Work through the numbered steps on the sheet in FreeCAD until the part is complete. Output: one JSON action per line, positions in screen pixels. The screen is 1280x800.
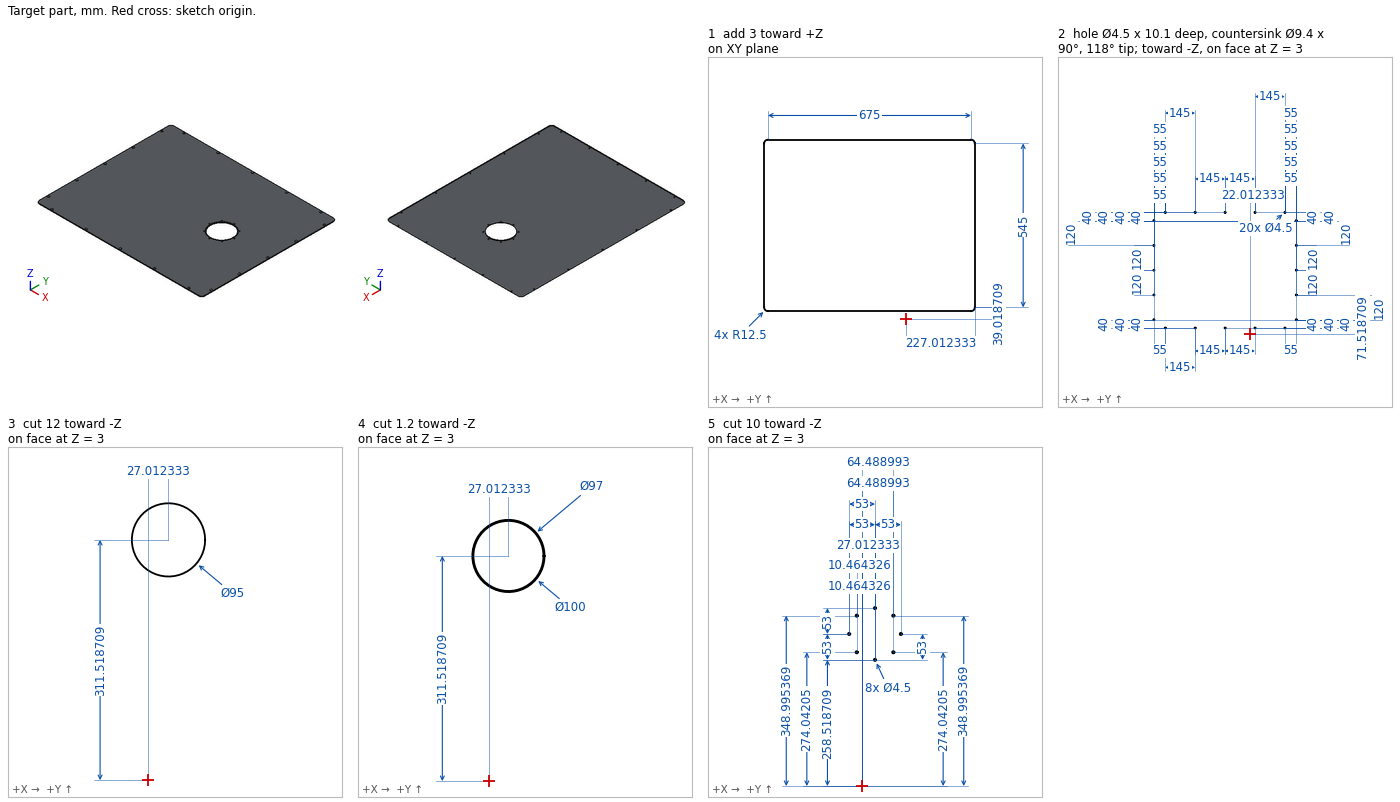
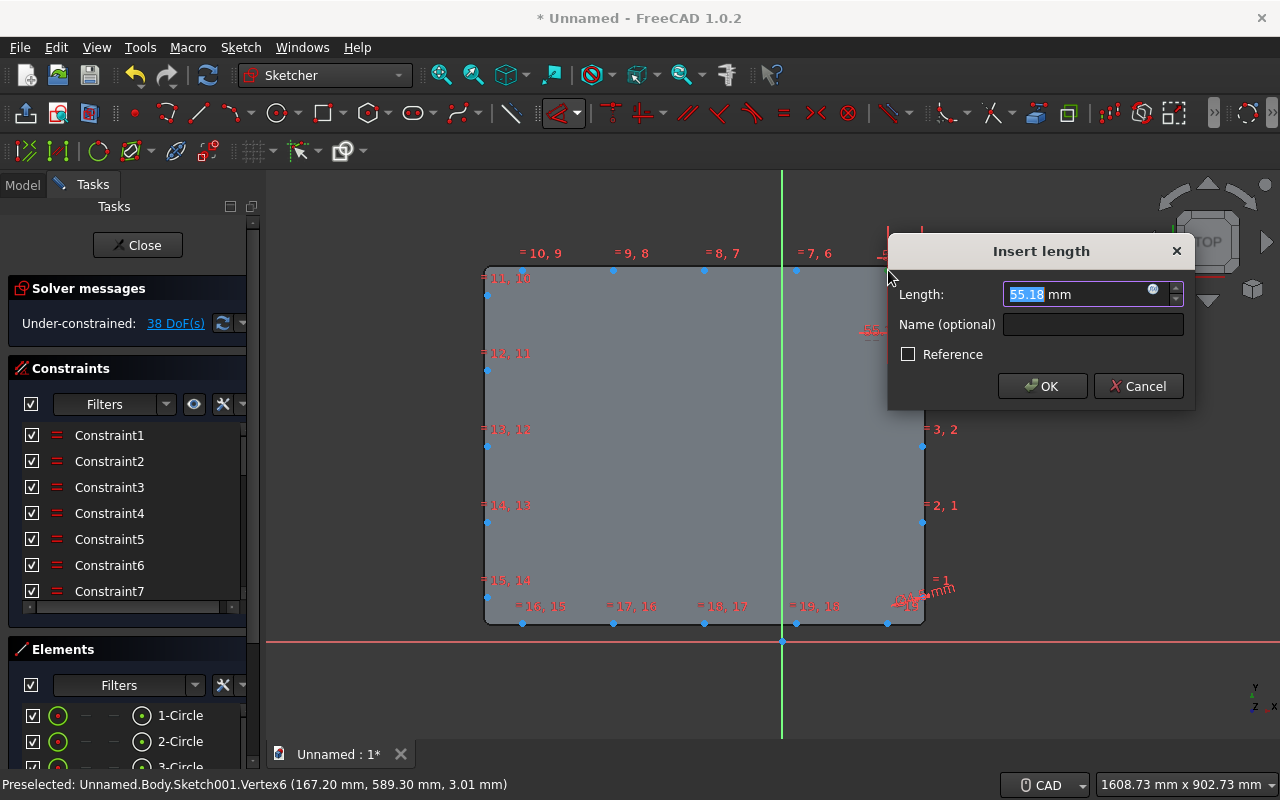
{"action": "type", "text": "55"}
{"action": "key", "text": "Return"}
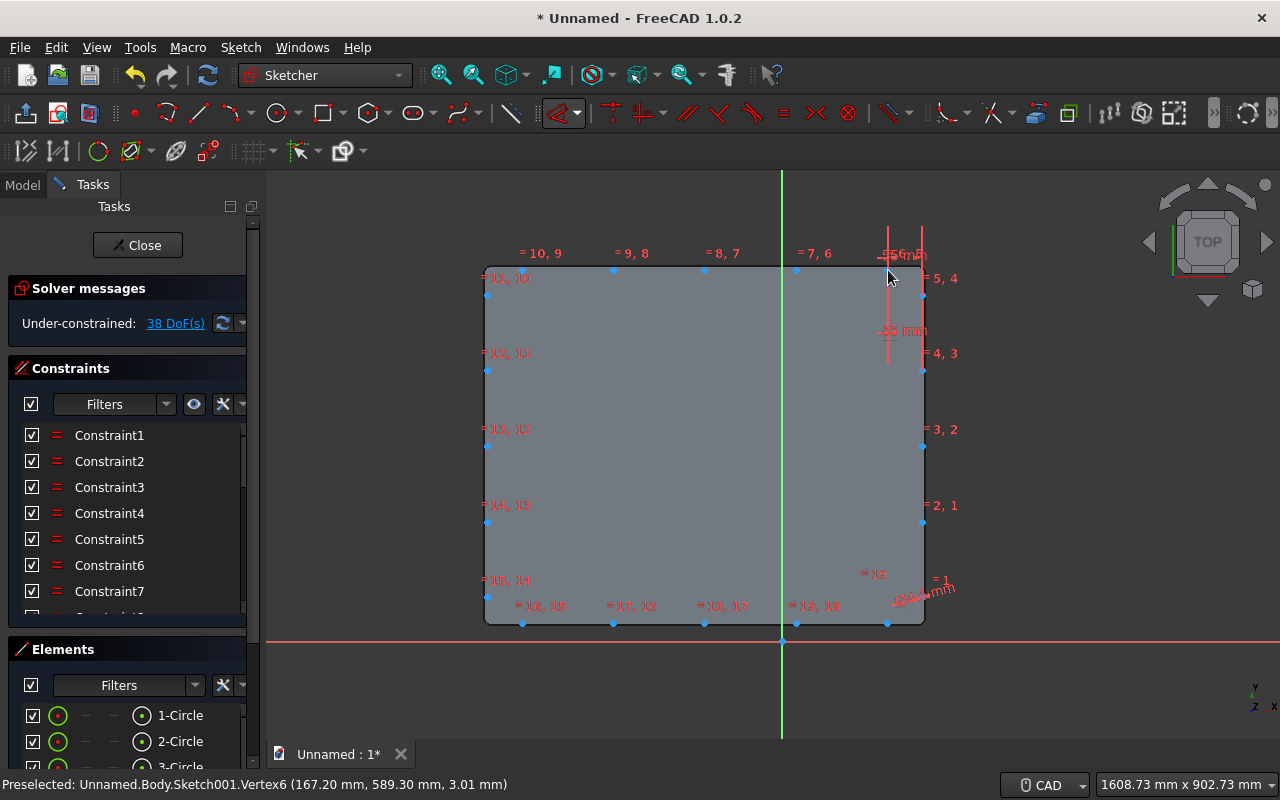
{"action": "left_click", "coordinate": [922, 446]}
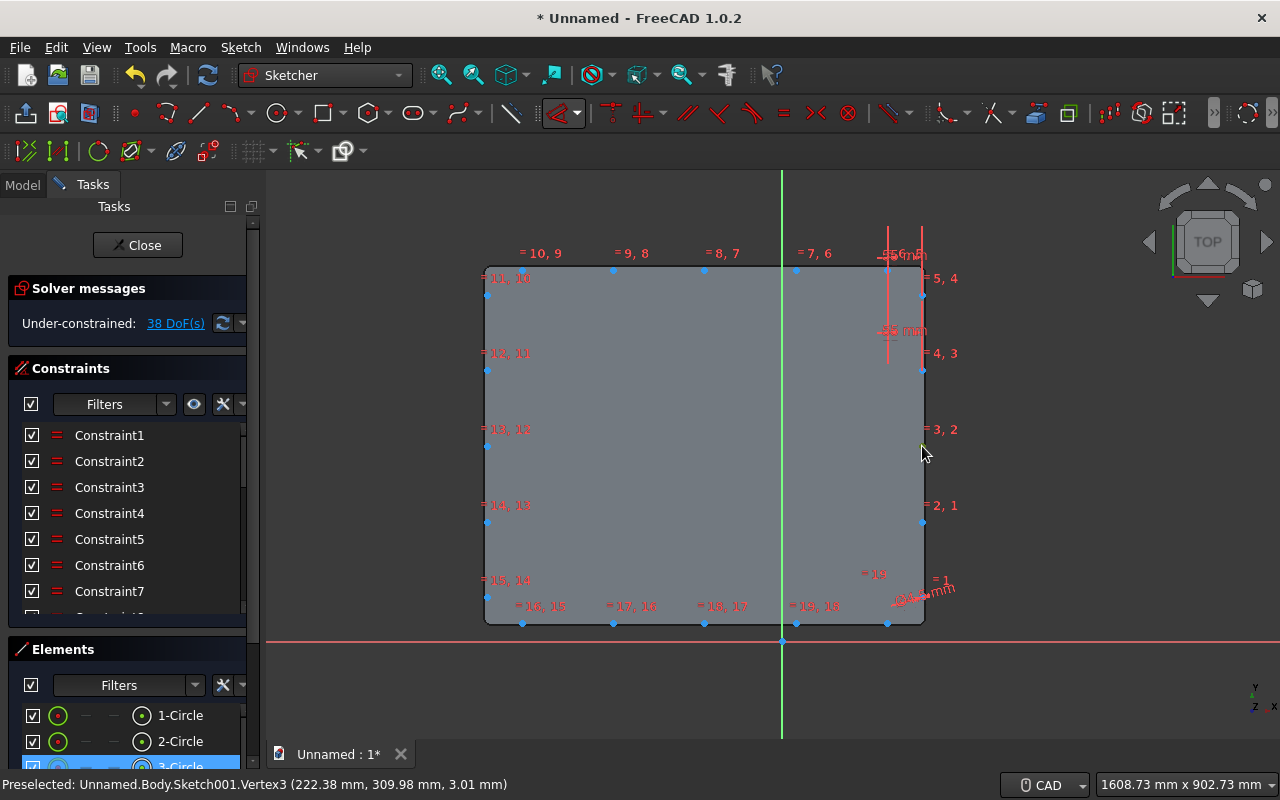
{"action": "left_click", "coordinate": [888, 270]}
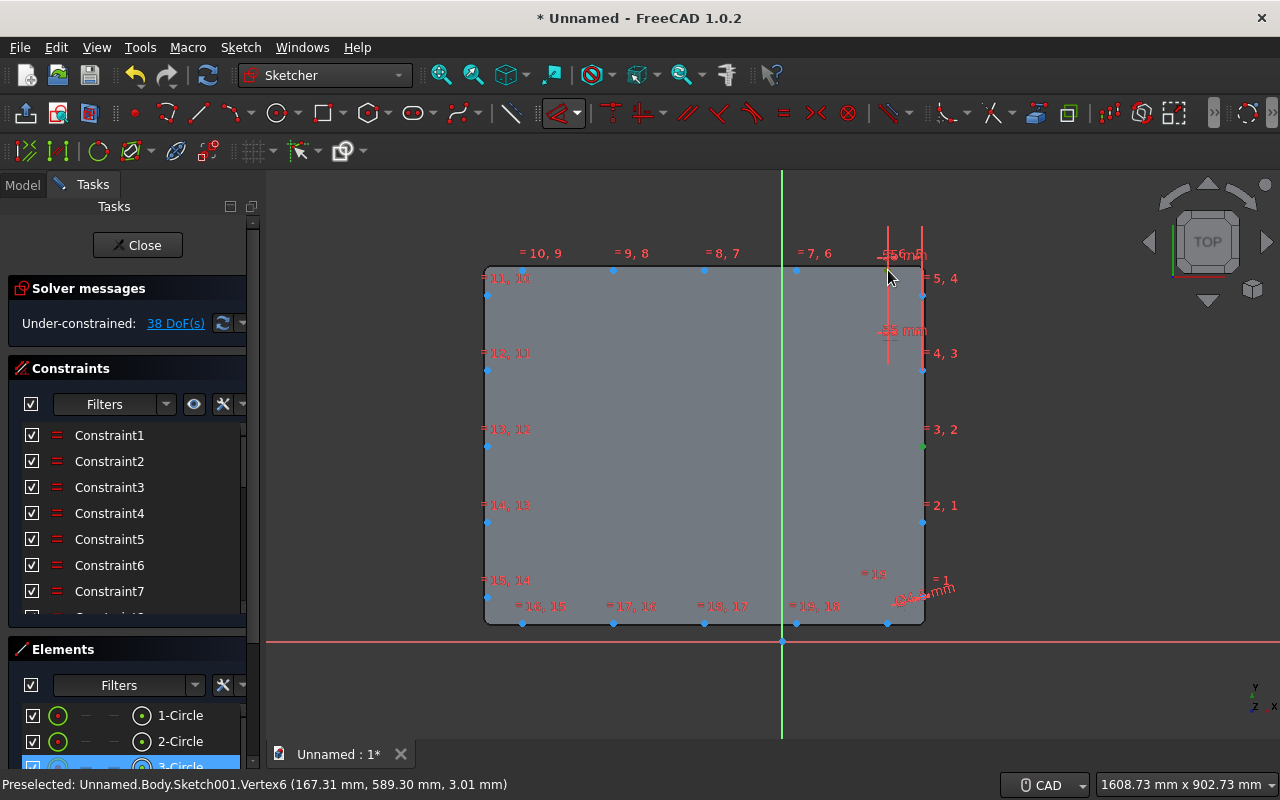
{"action": "key", "text": "l"}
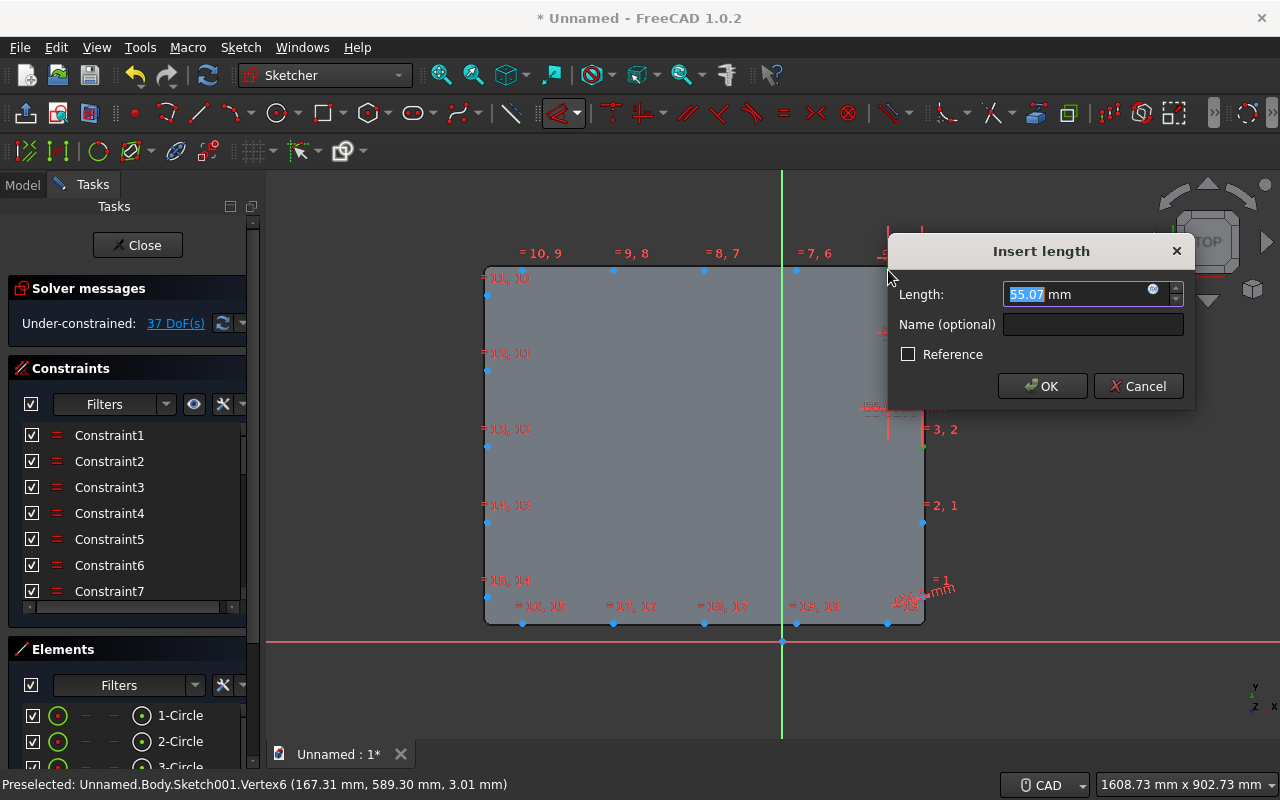
{"action": "type", "text": "55"}
{"action": "key", "text": "Return"}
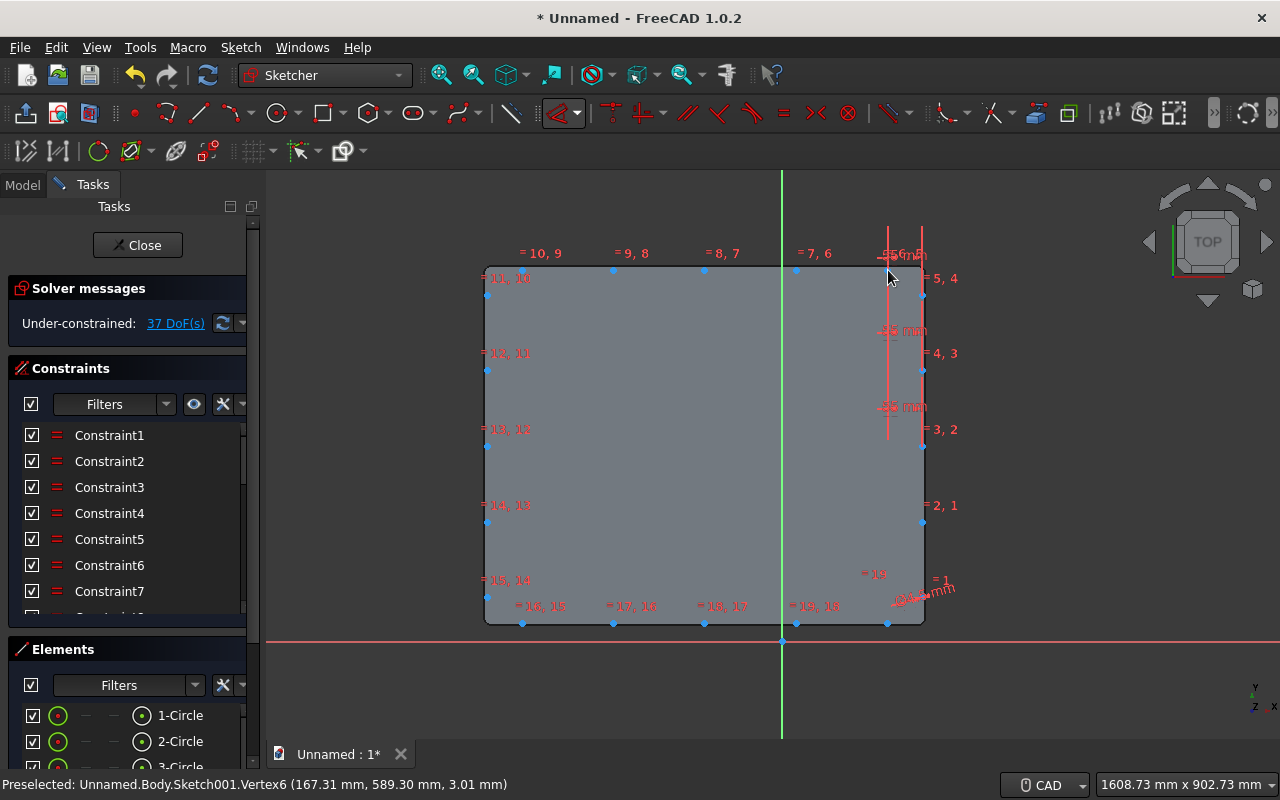
{"action": "left_click", "coordinate": [922, 522]}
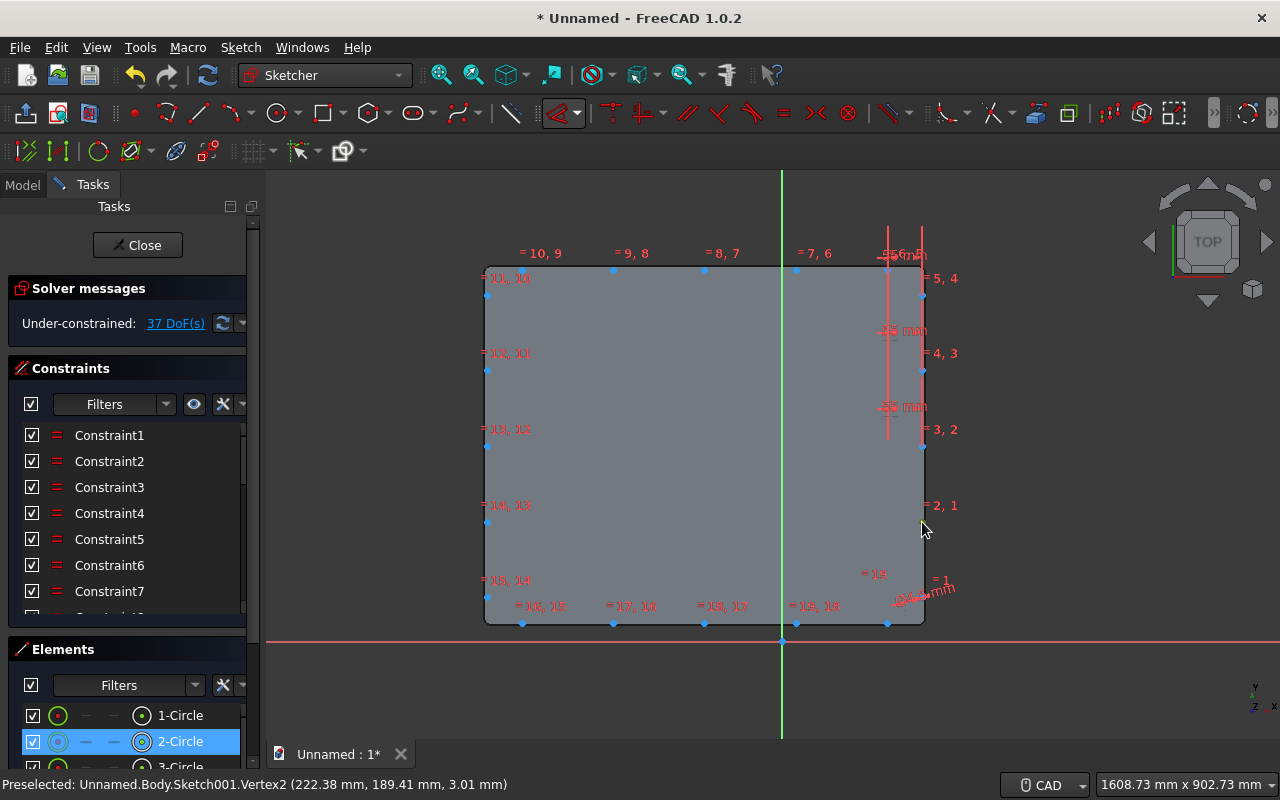
{"action": "left_click", "coordinate": [888, 270]}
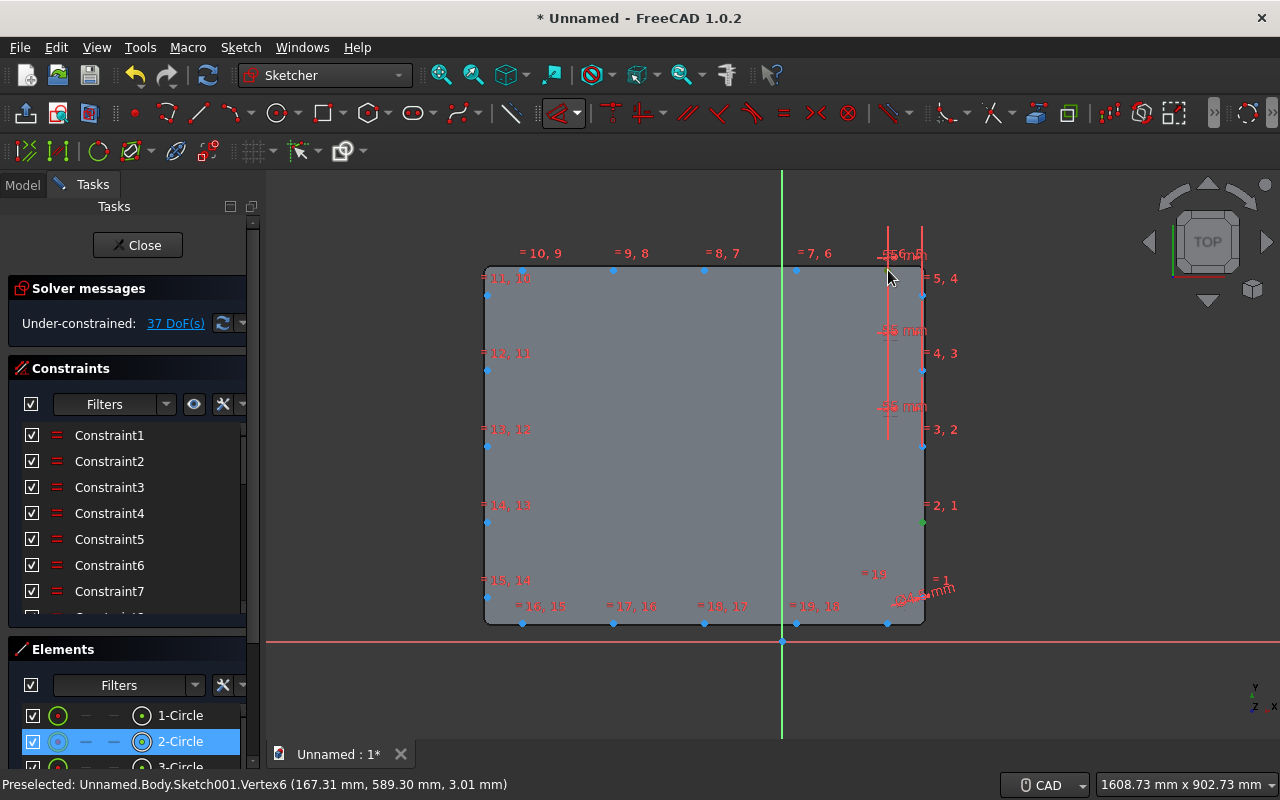
{"action": "key", "text": "l"}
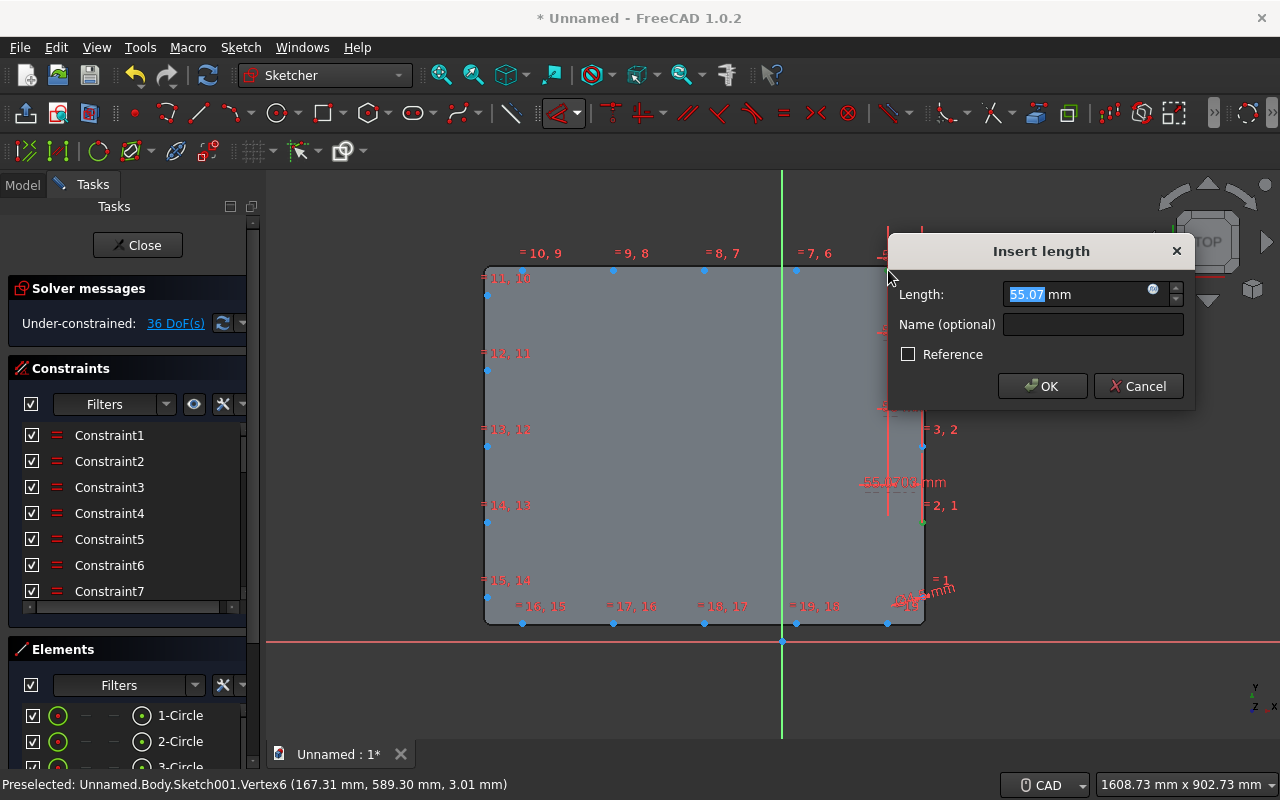
{"action": "type", "text": "55"}
{"action": "key", "text": "Return"}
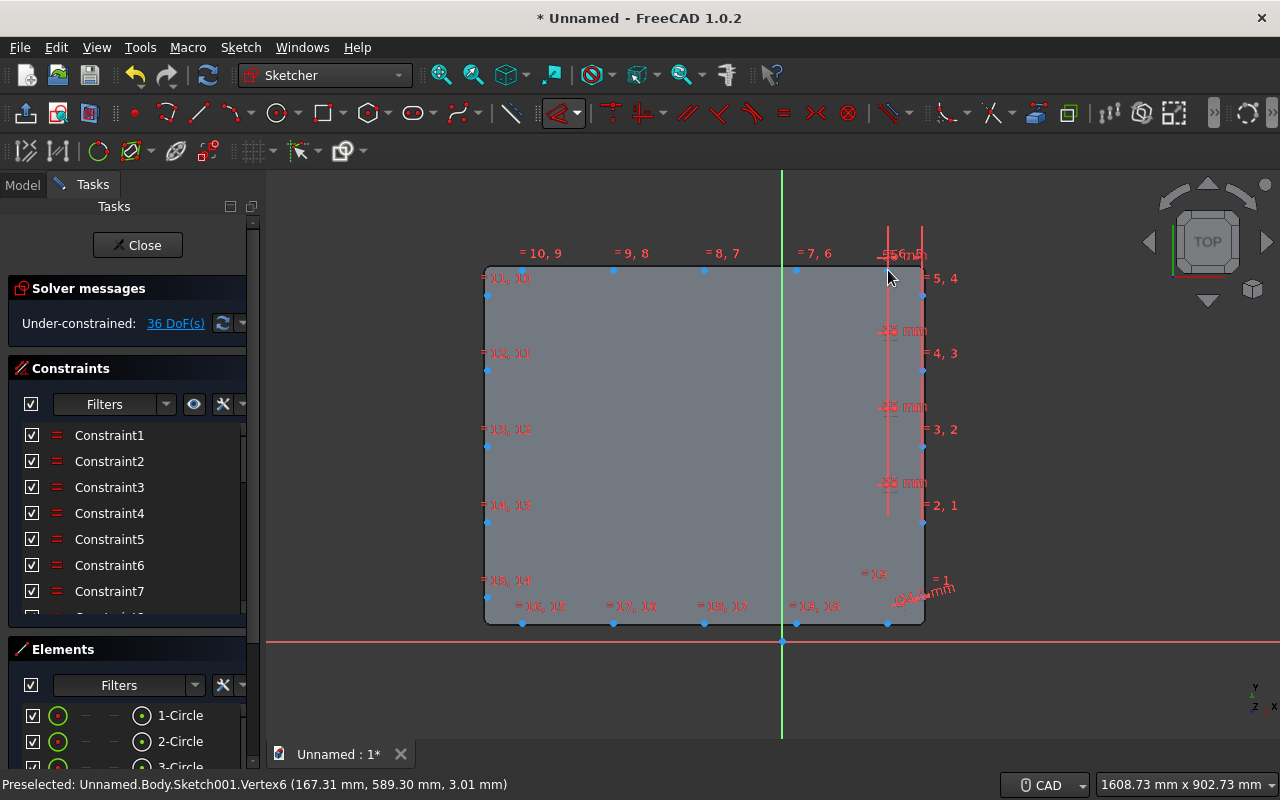
{"action": "left_click", "coordinate": [922, 597]}